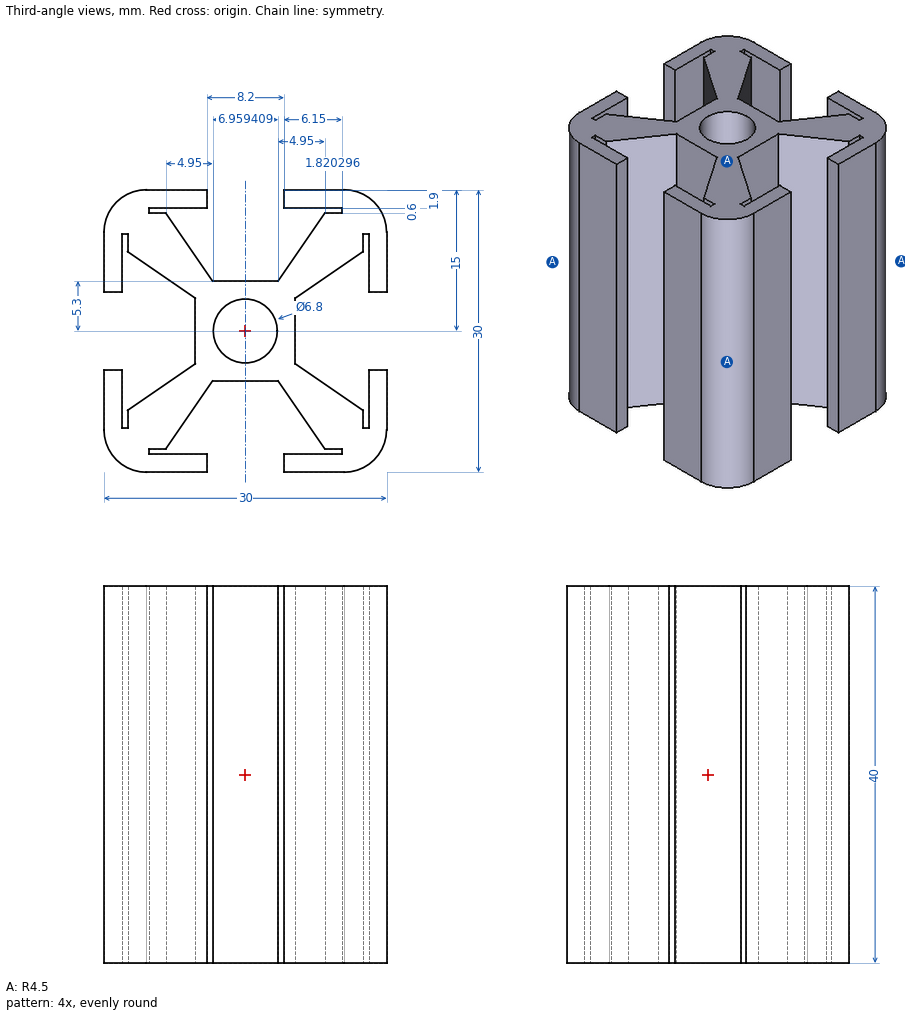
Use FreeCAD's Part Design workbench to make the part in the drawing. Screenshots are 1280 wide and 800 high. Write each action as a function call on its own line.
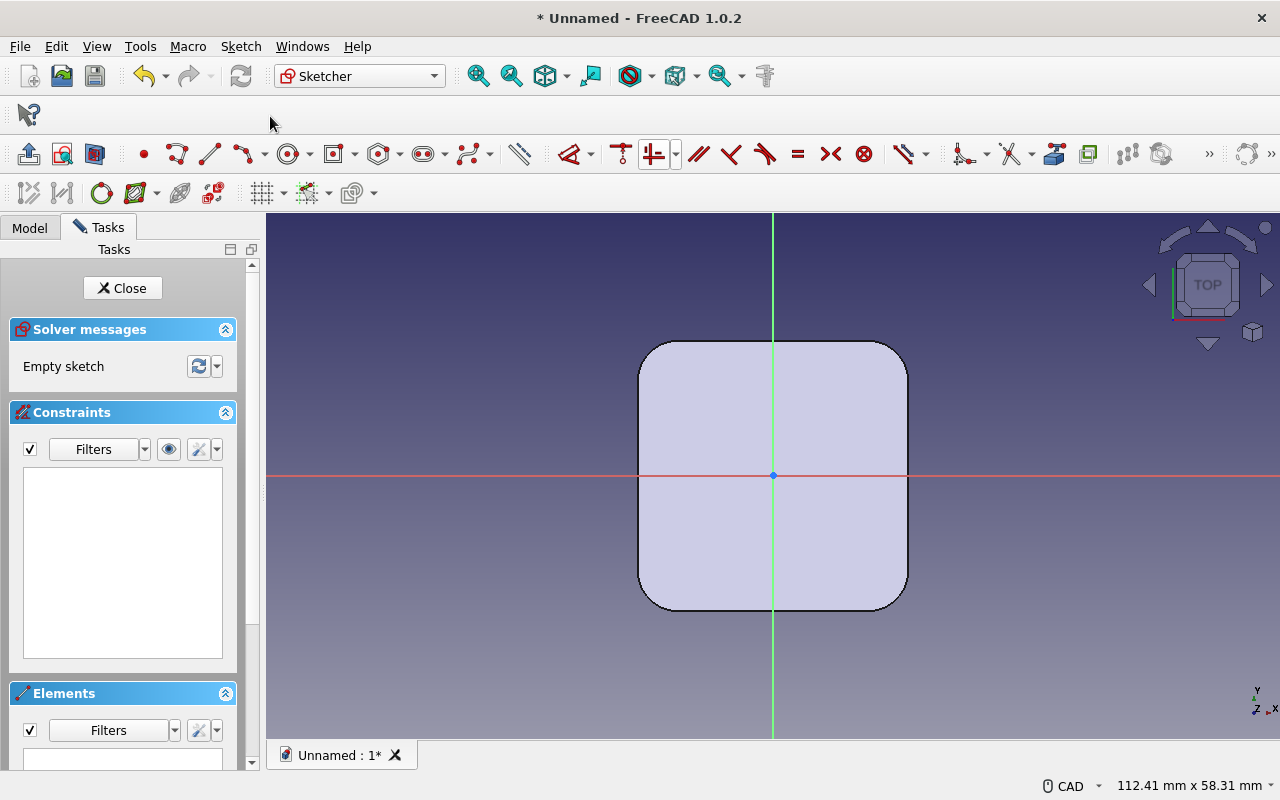
scroll(856, 360, up, 3)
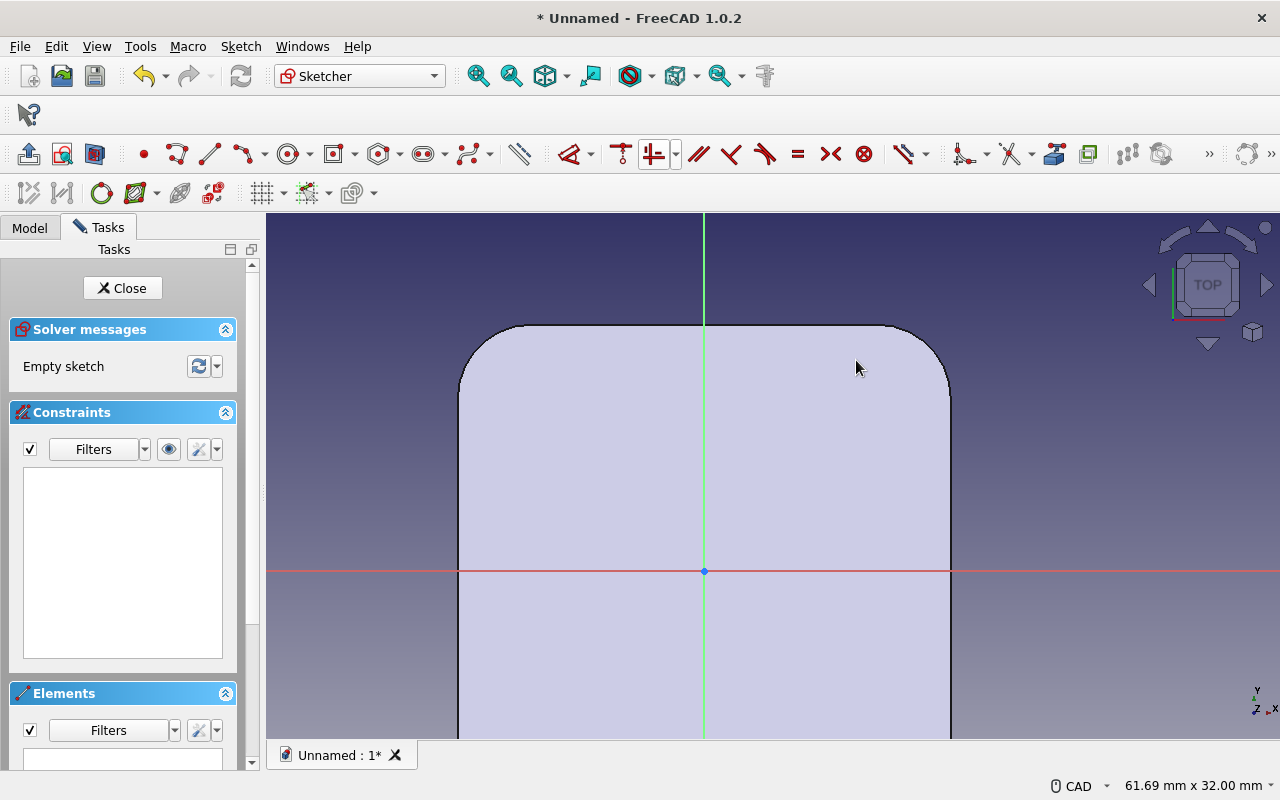
key(g)
key(m)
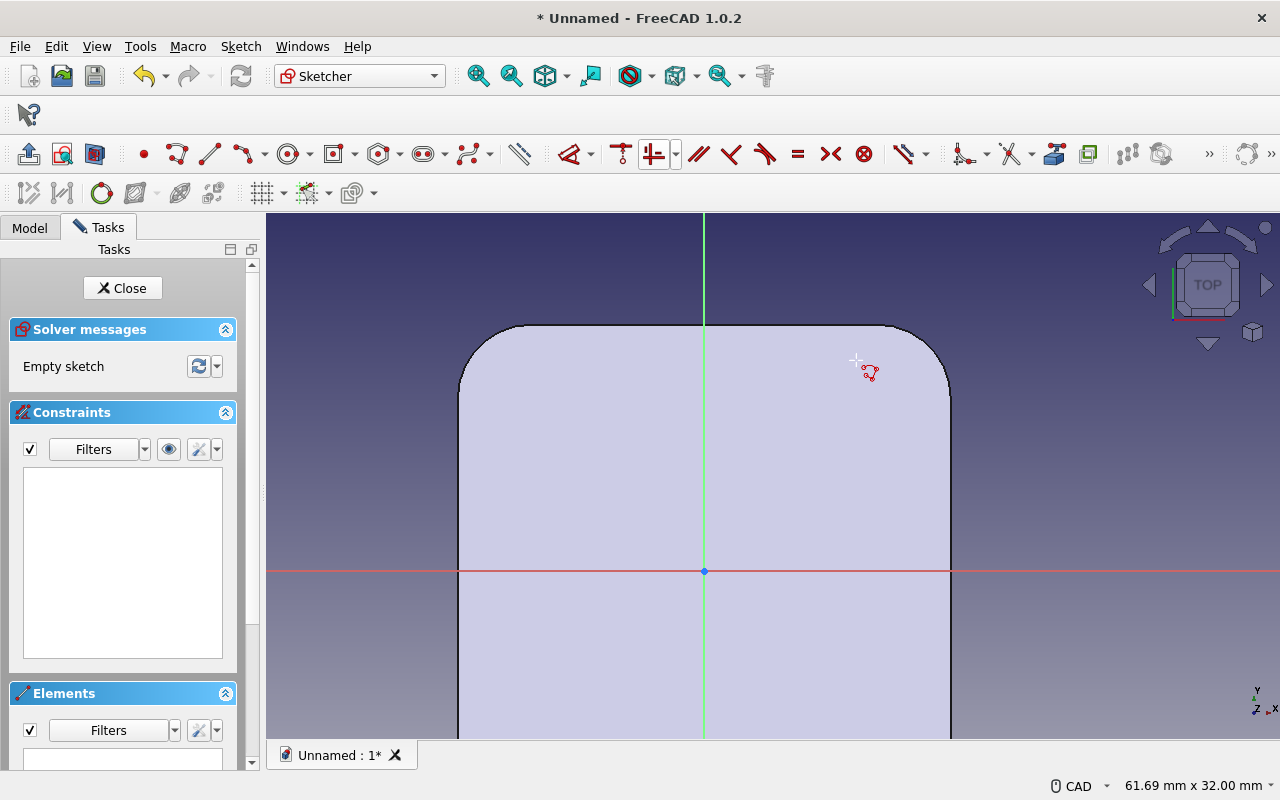
click(647, 484)
click(761, 484)
click(843, 366)
click(873, 366)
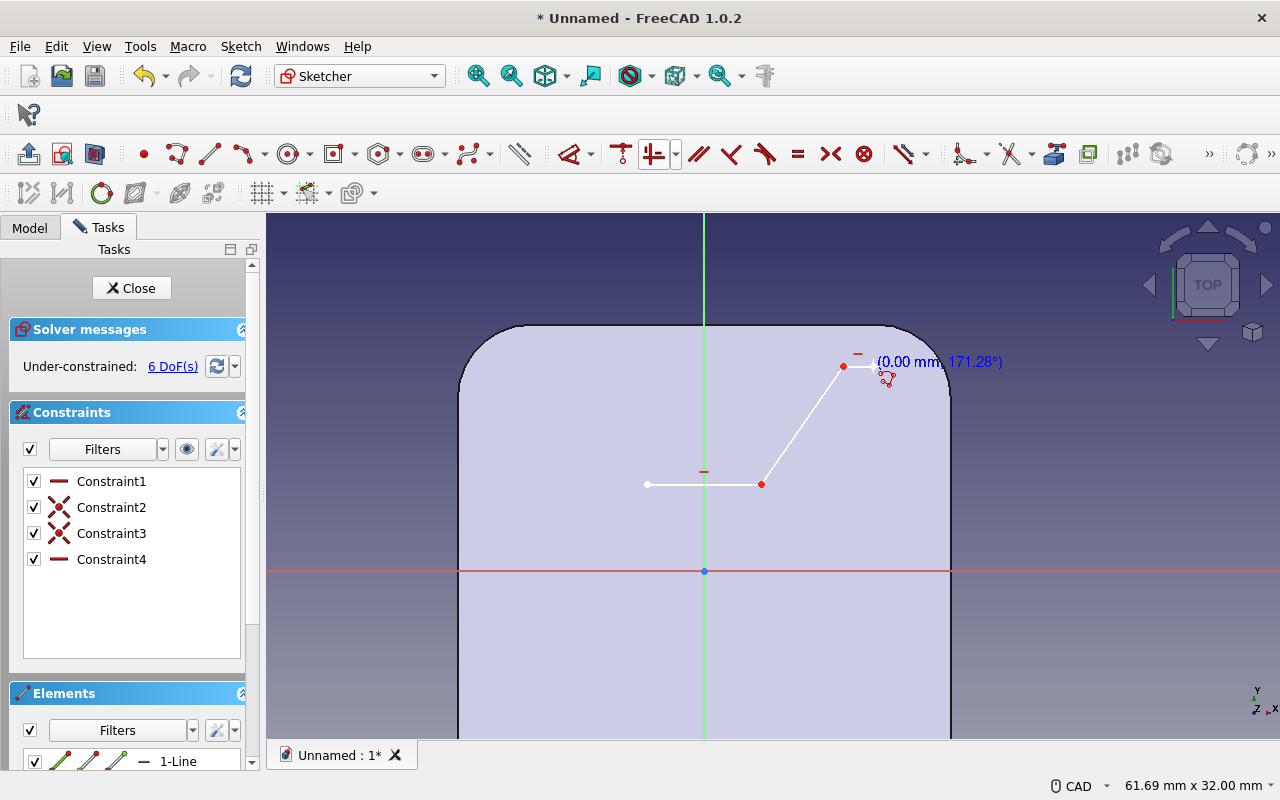
scroll(873, 356, up, 3)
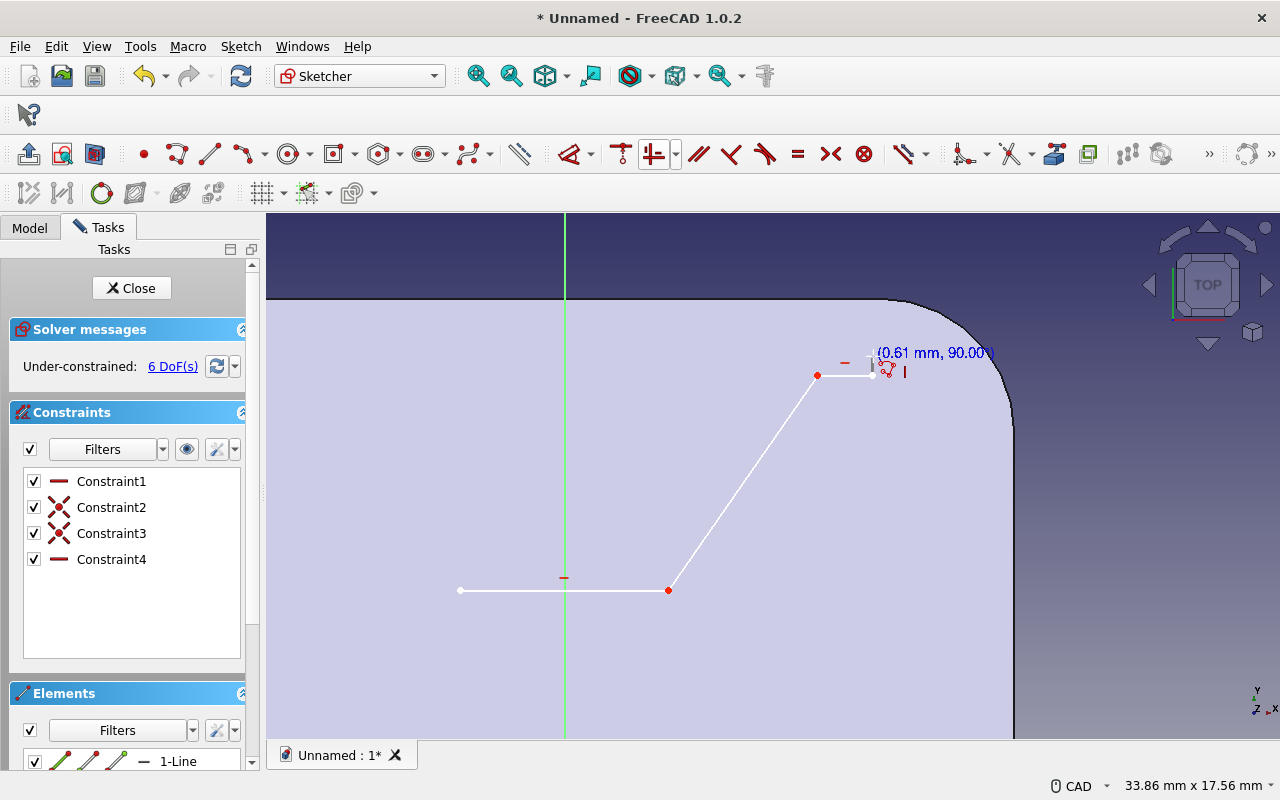
click(873, 355)
click(688, 355)
click(688, 299)
click(442, 299)
click(442, 355)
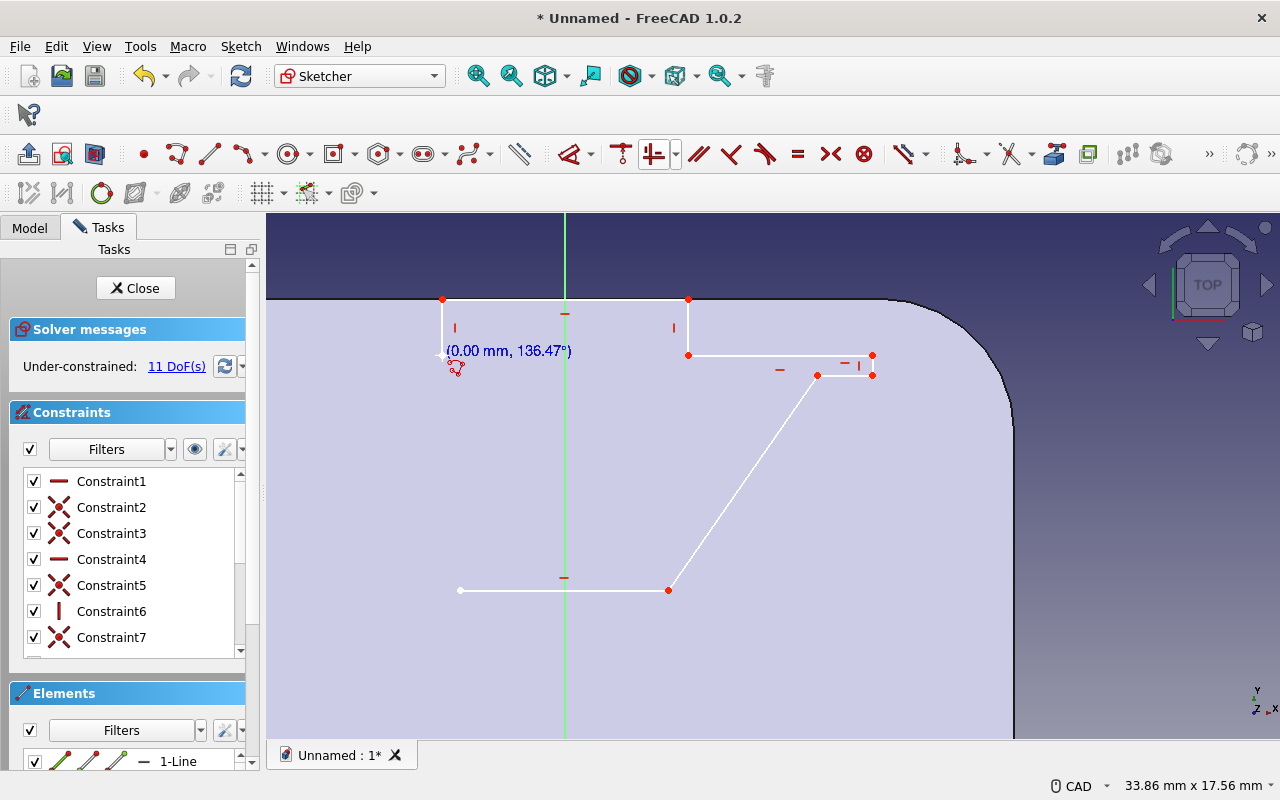
scroll(874, 357, down, 3)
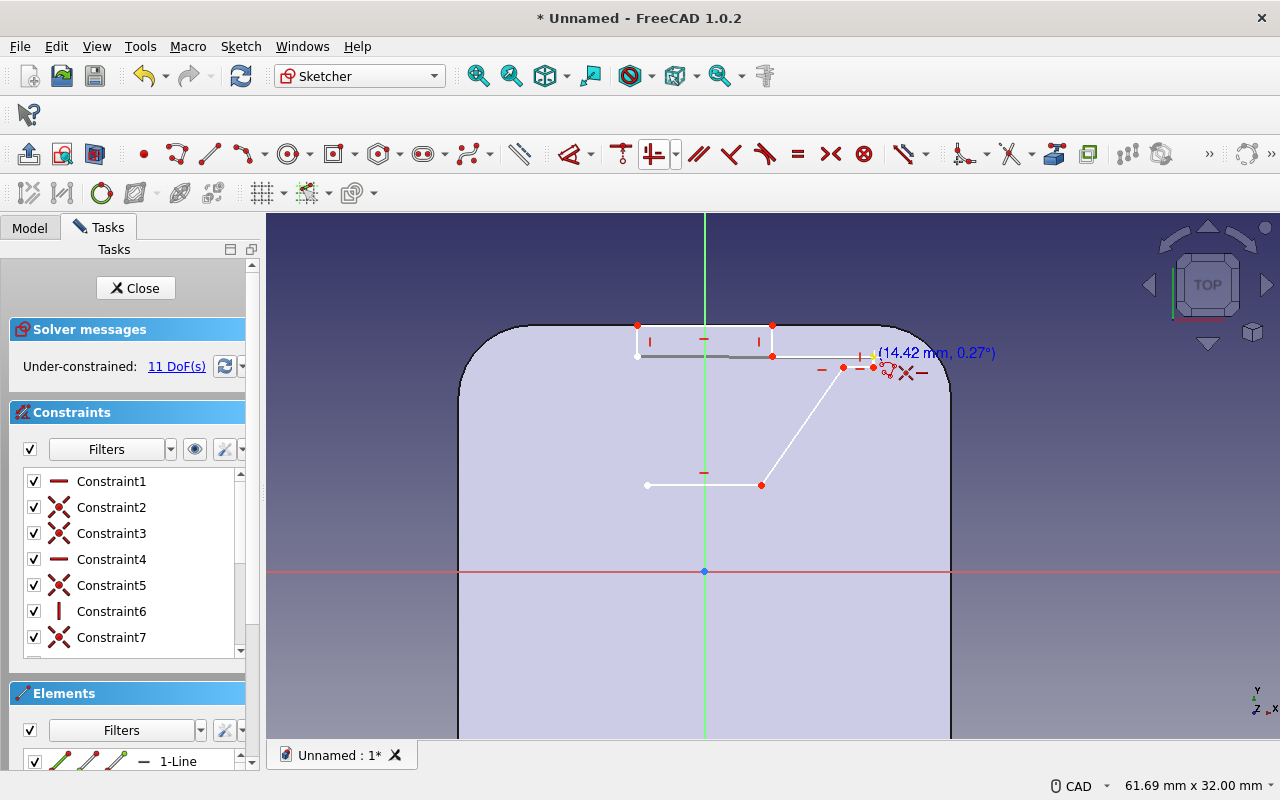
click(536, 356)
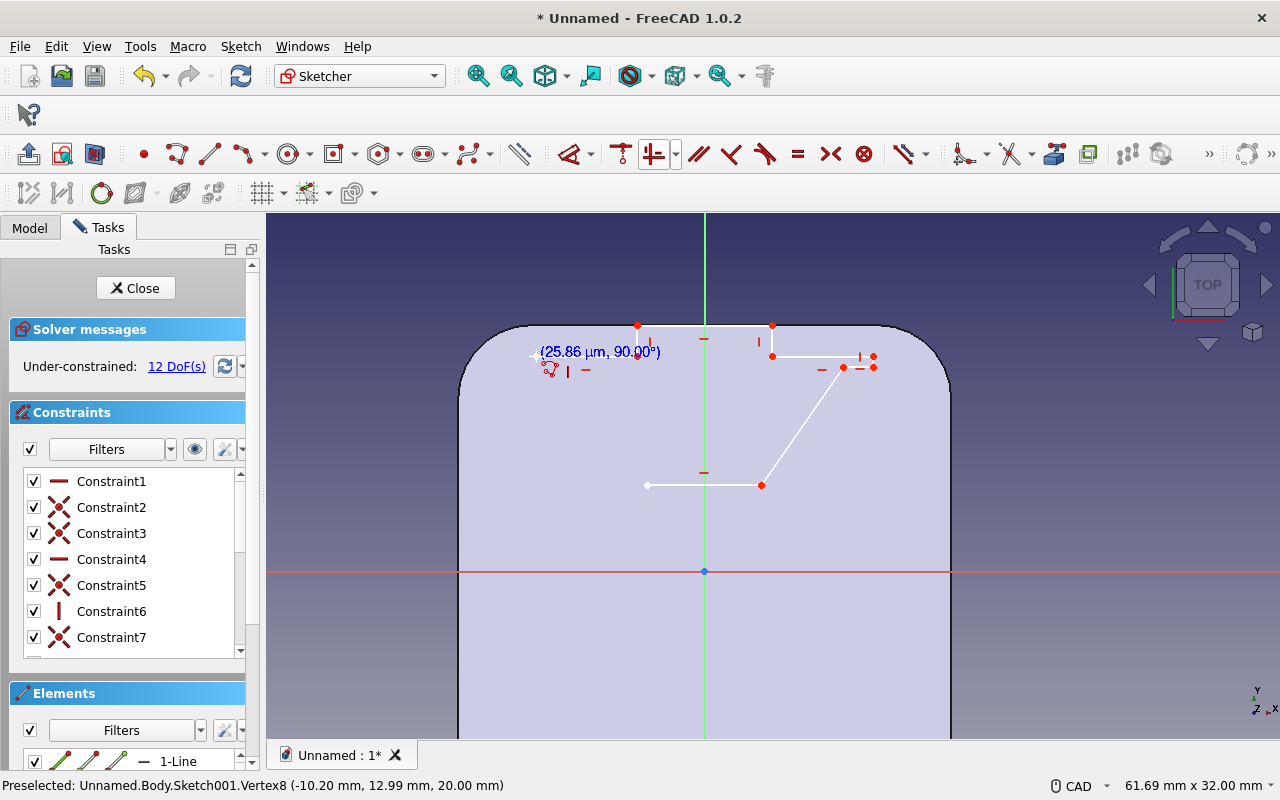
scroll(536, 366, up, 3)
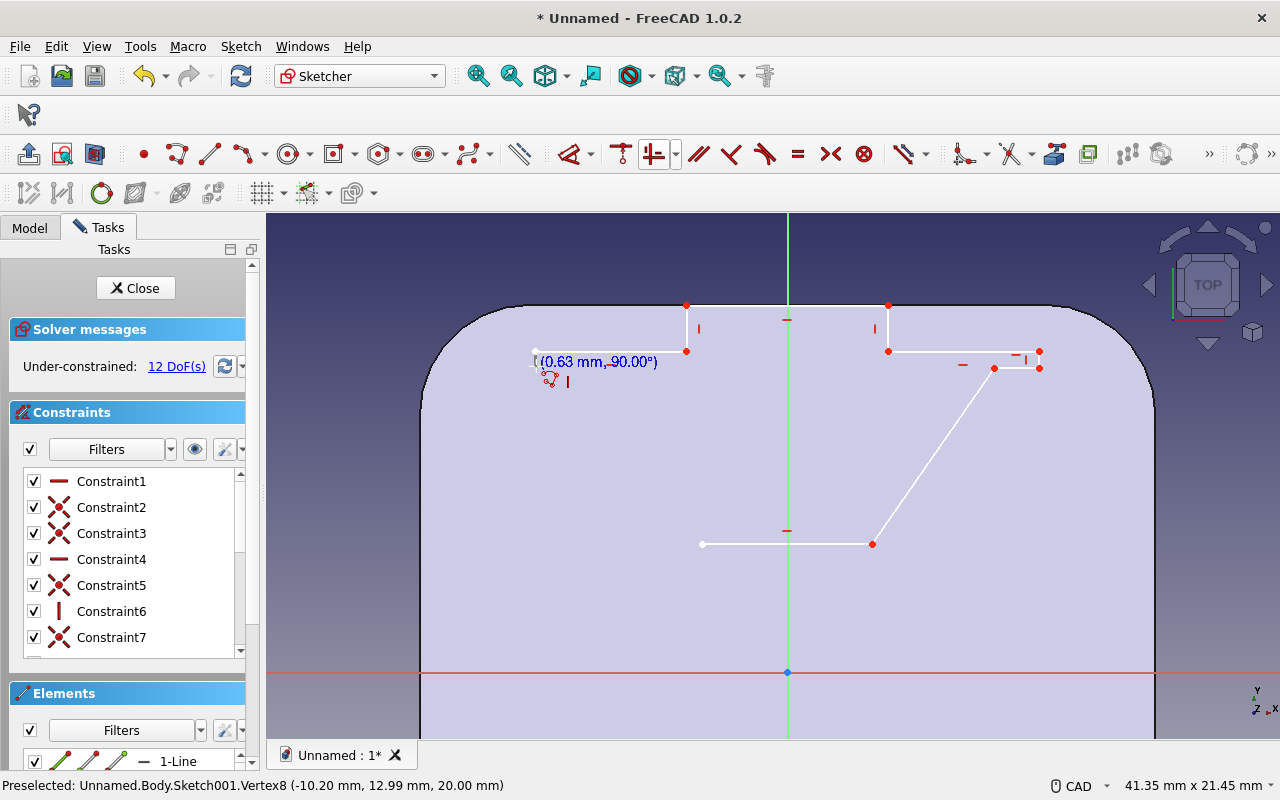
click(536, 366)
click(591, 366)
click(739, 583)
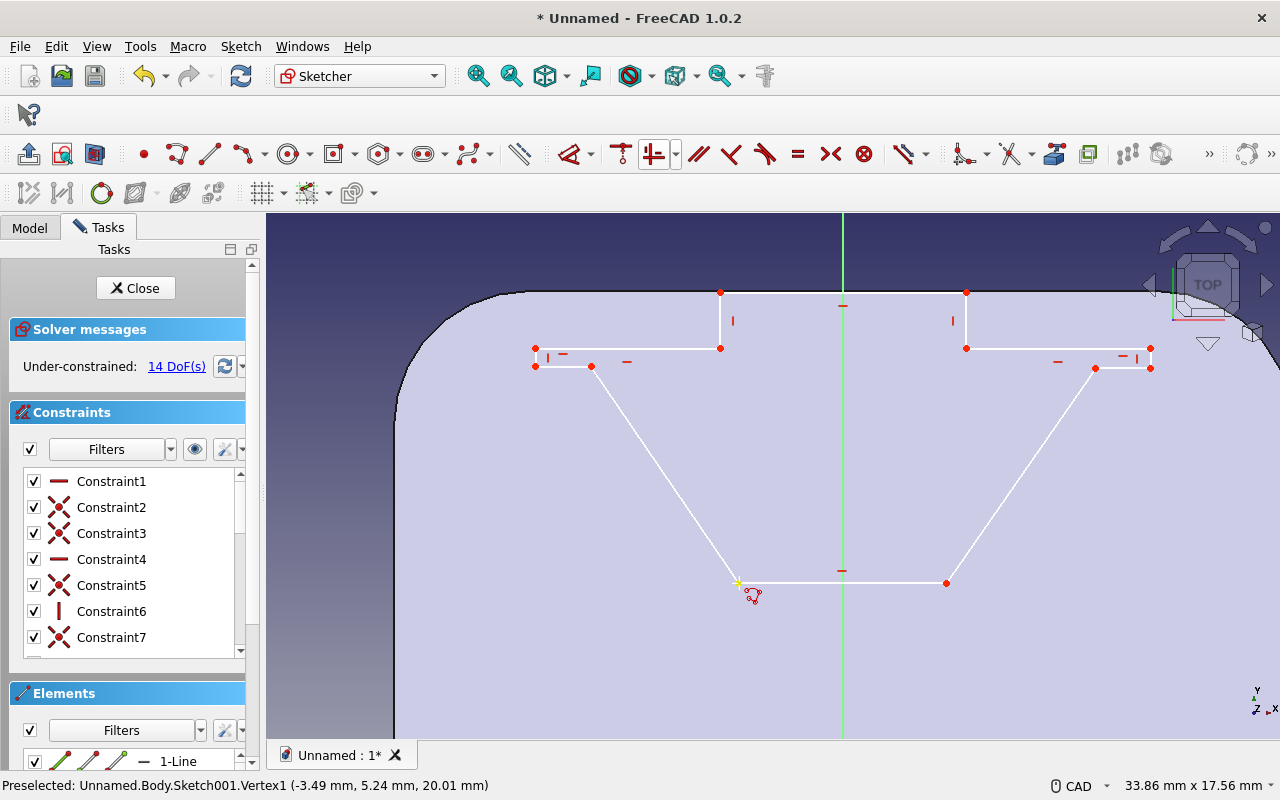
key(g)
key(c)